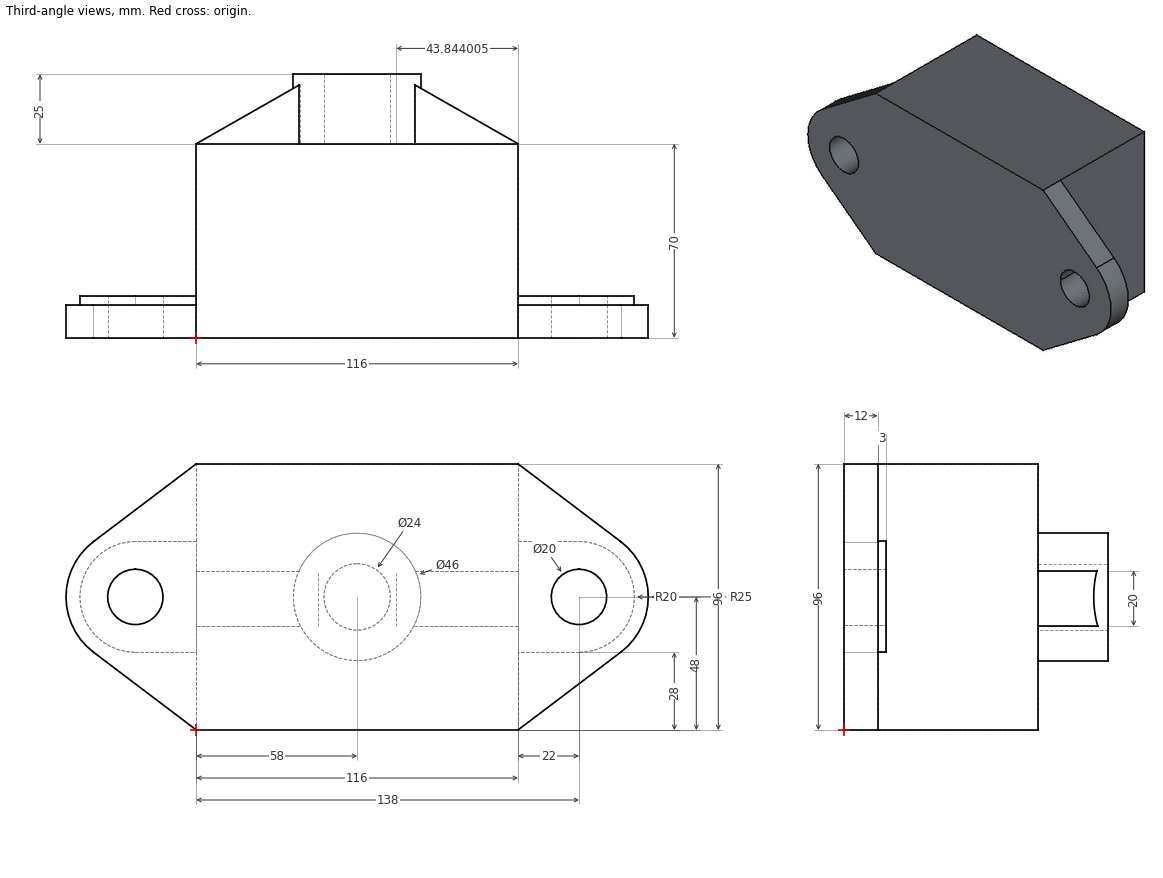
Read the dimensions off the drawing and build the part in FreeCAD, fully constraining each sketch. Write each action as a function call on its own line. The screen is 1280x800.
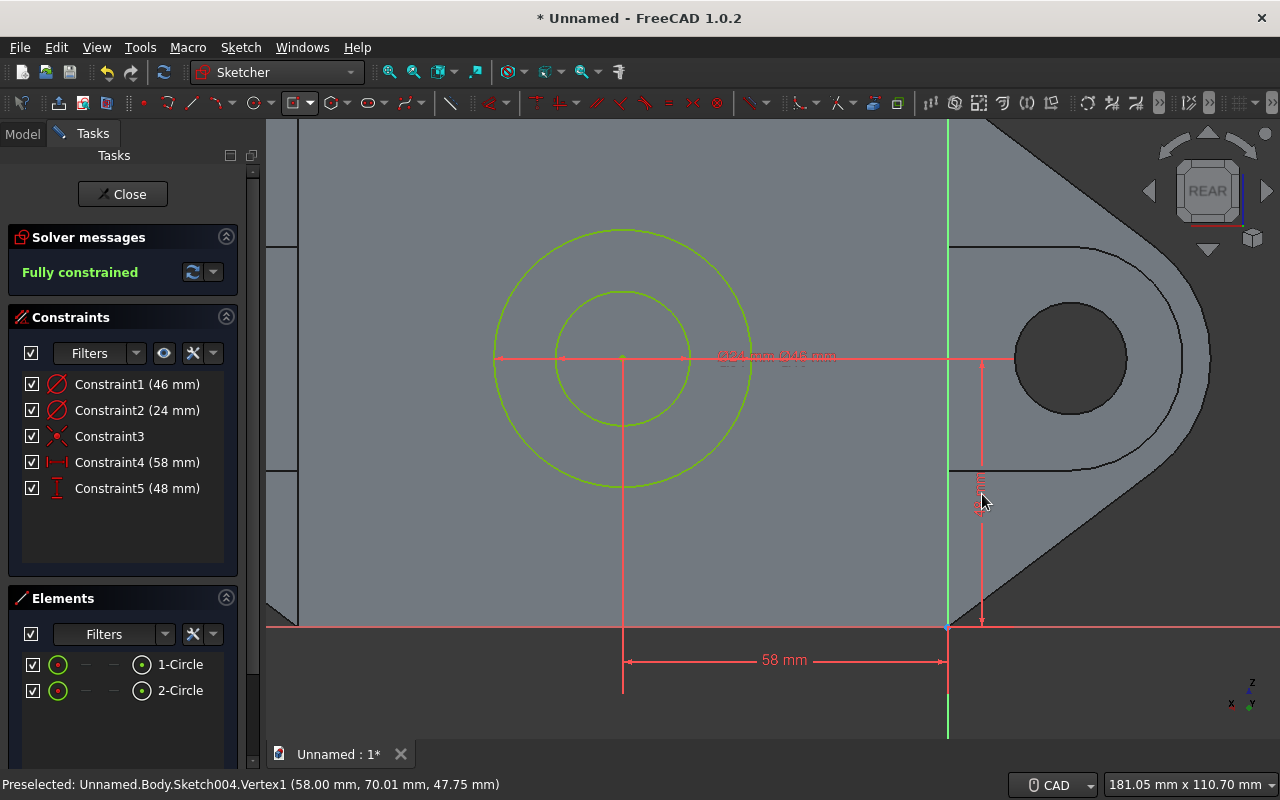
click(123, 194)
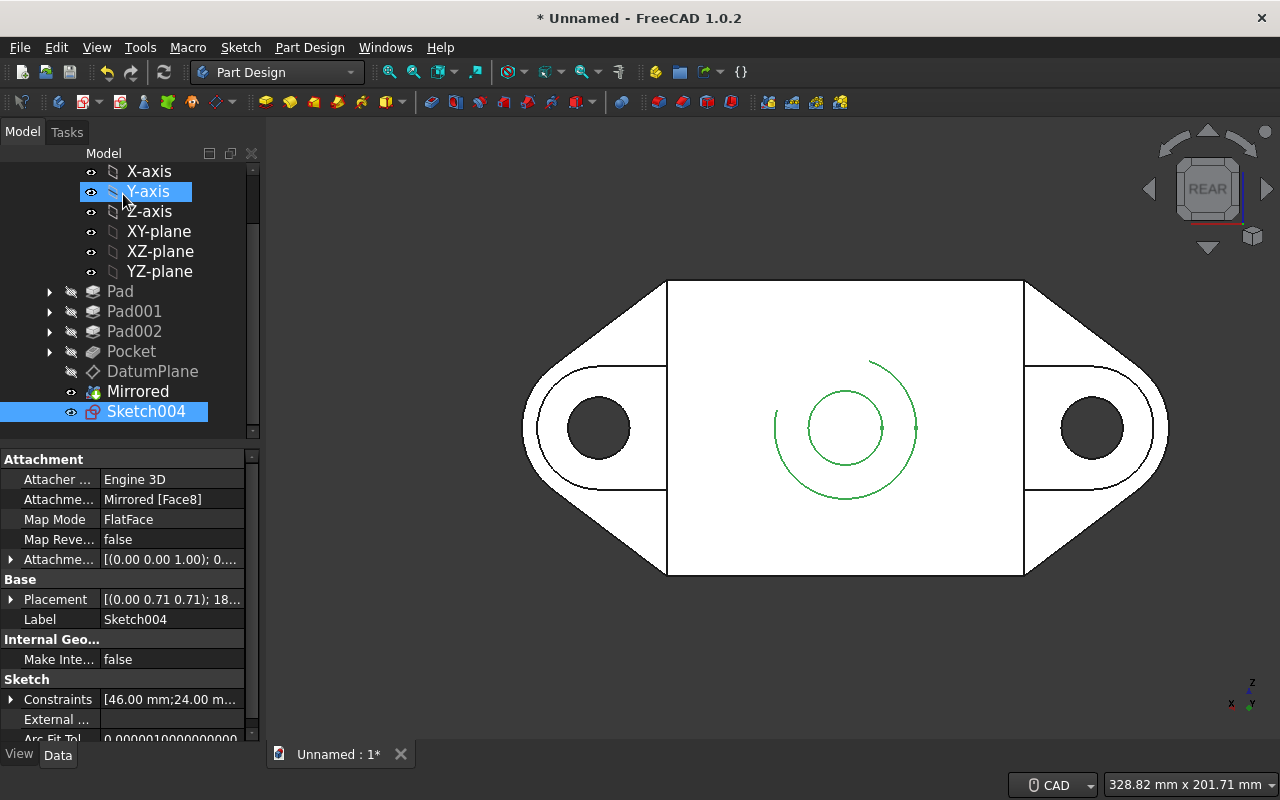
click(266, 102)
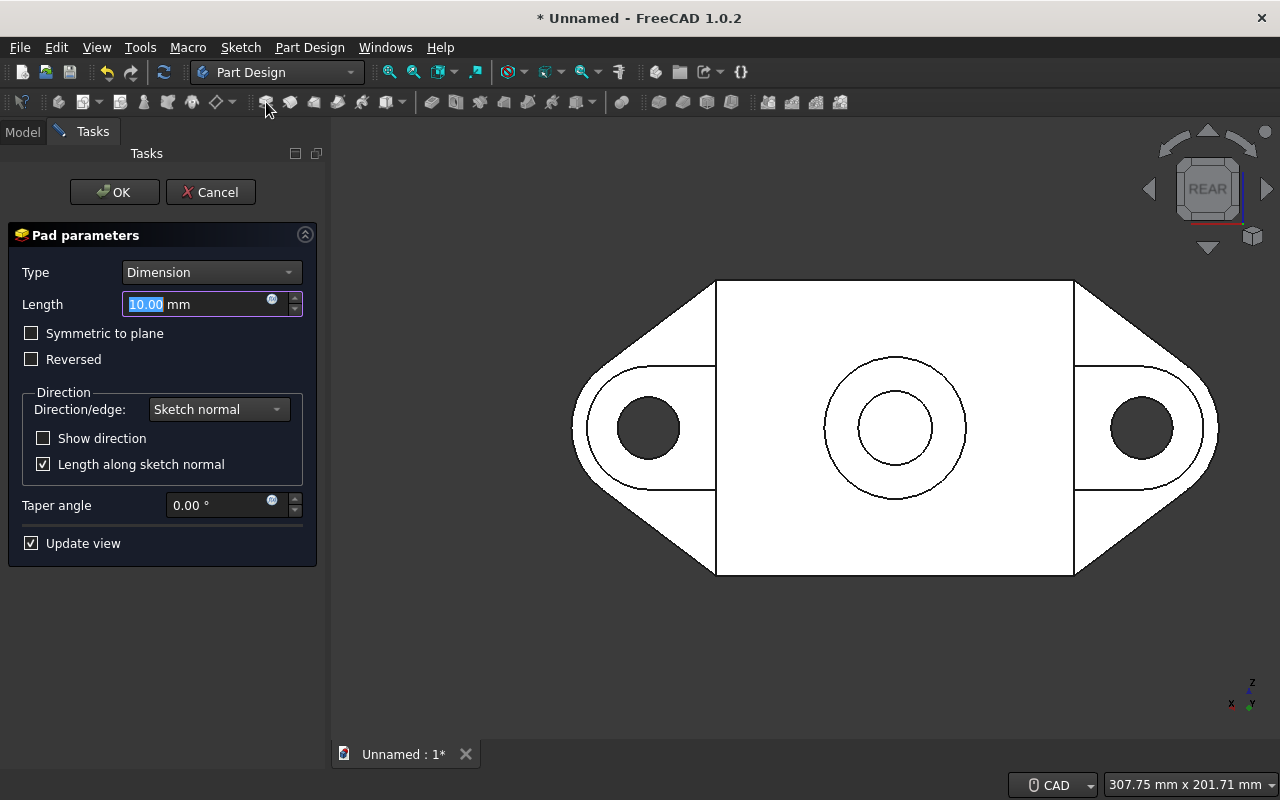
text(25)
key(Tab)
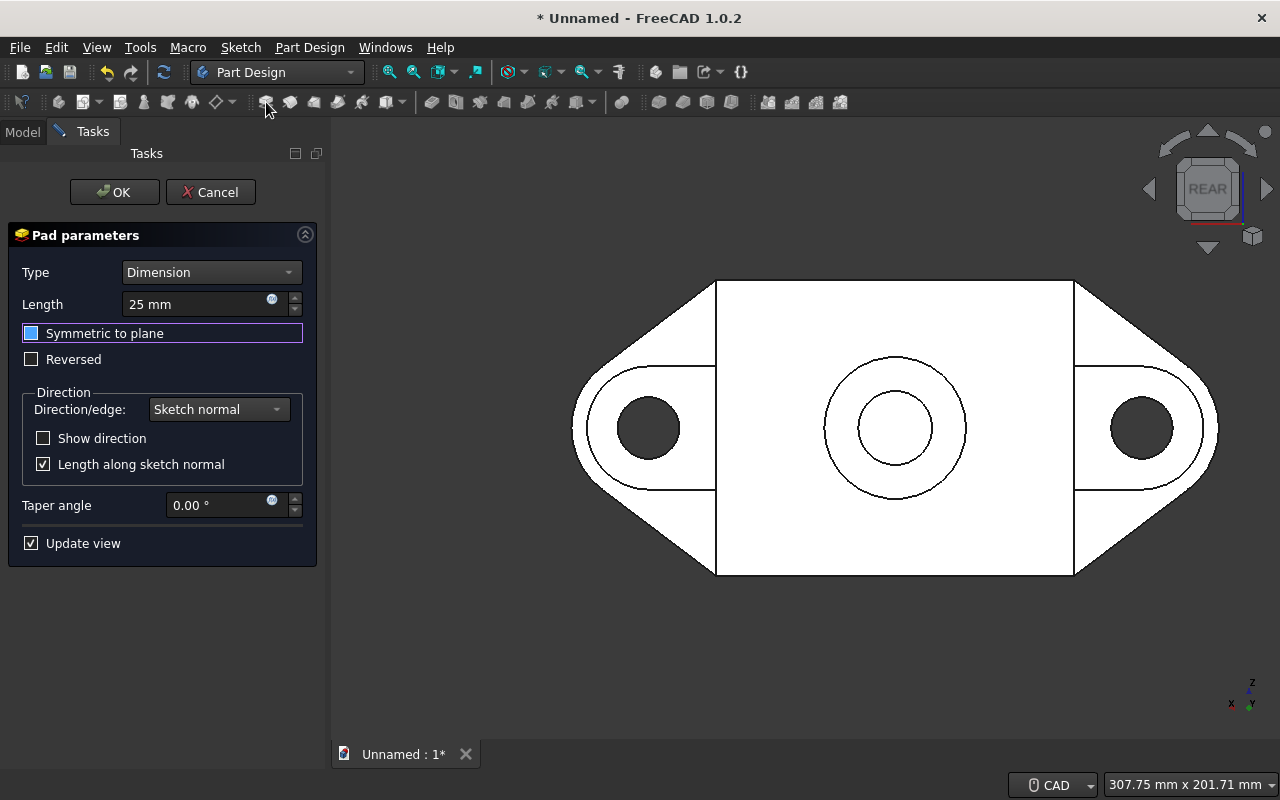
click(115, 192)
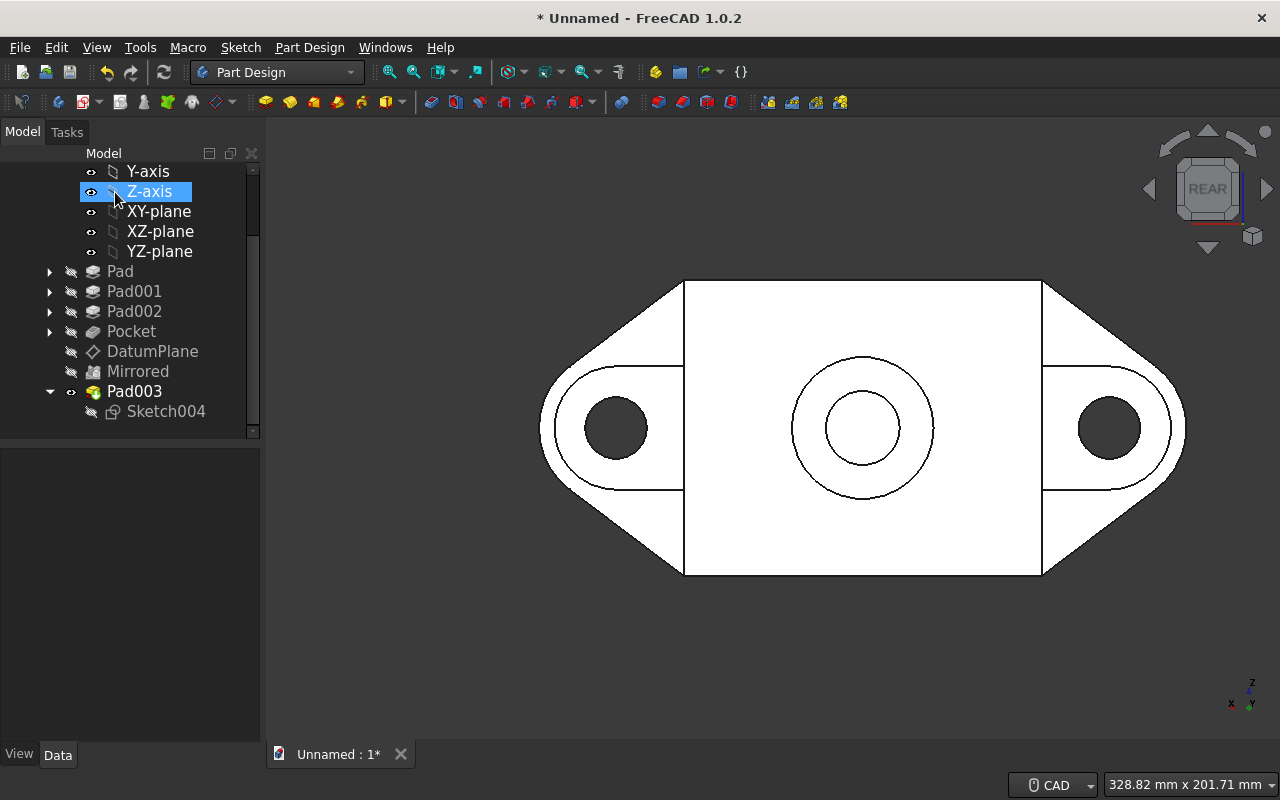
scroll(160, 287, down, 3)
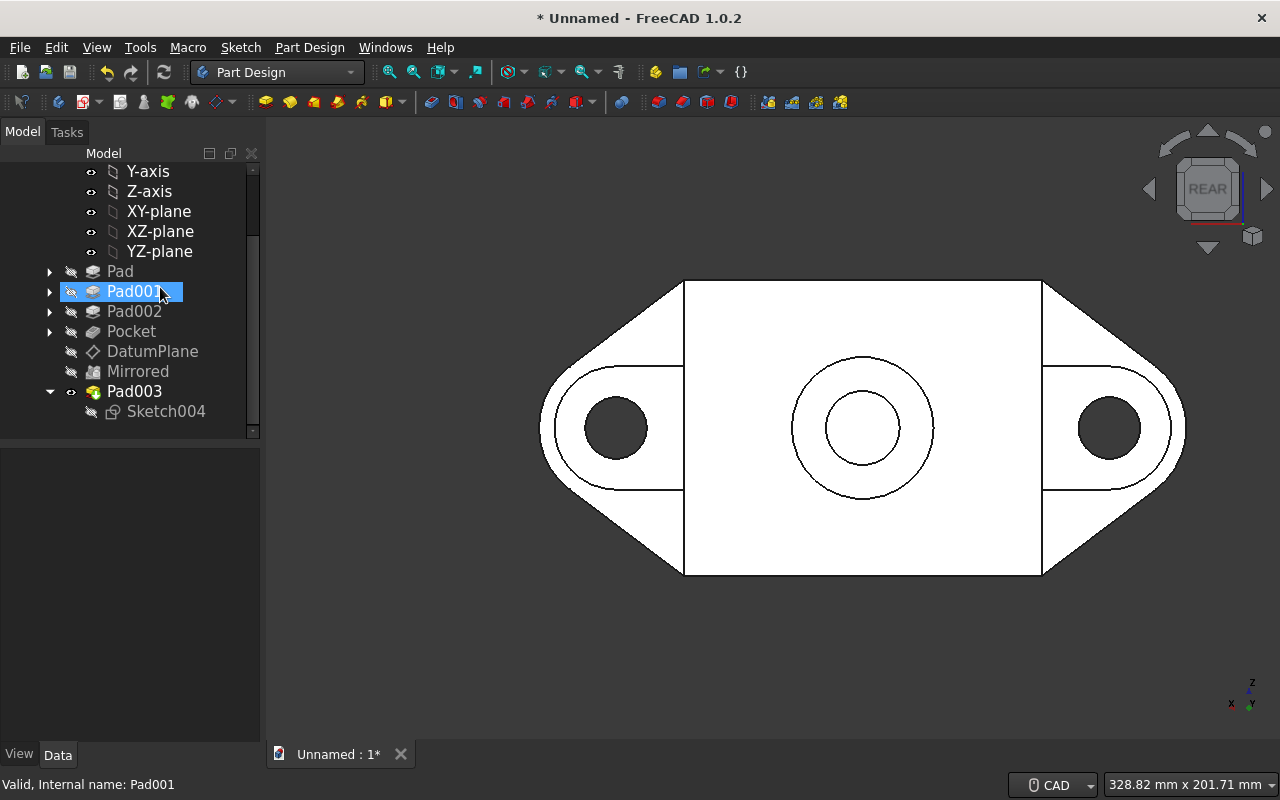
scroll(160, 287, up, 15)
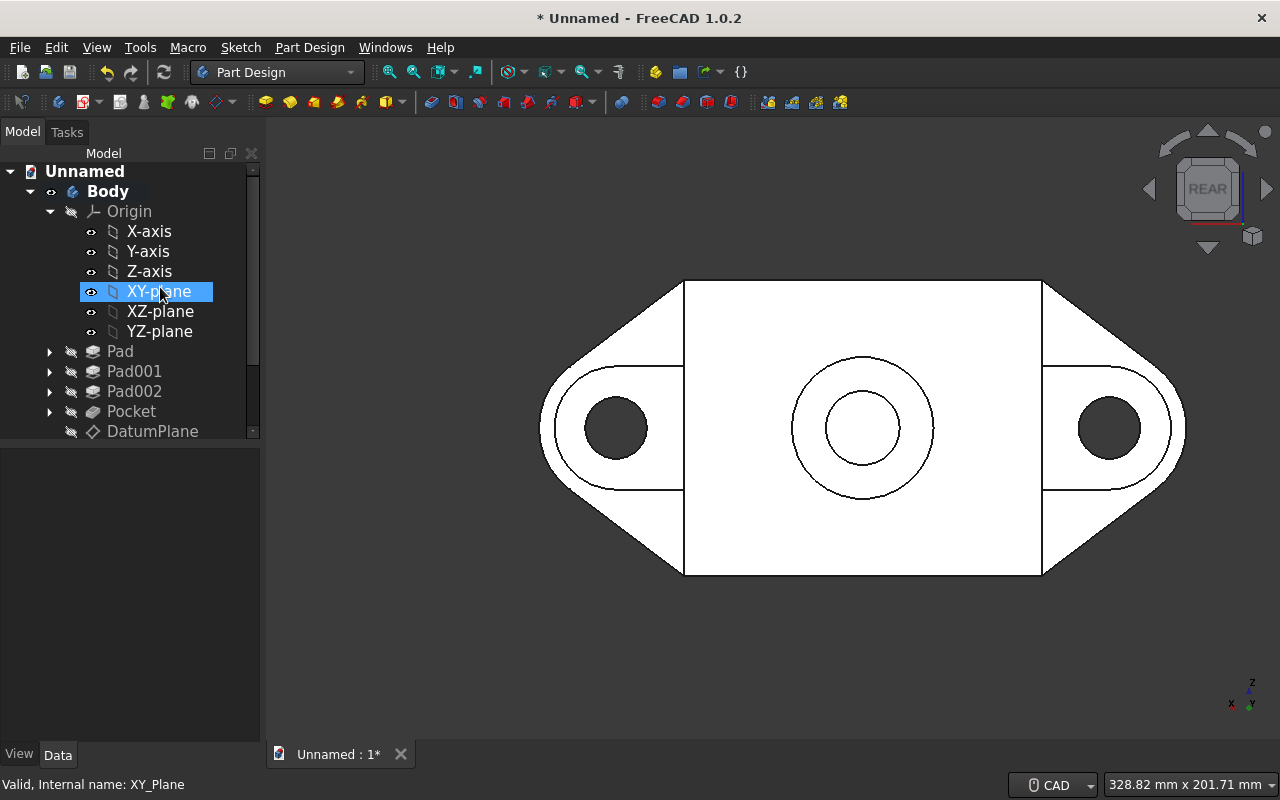
click(136, 292)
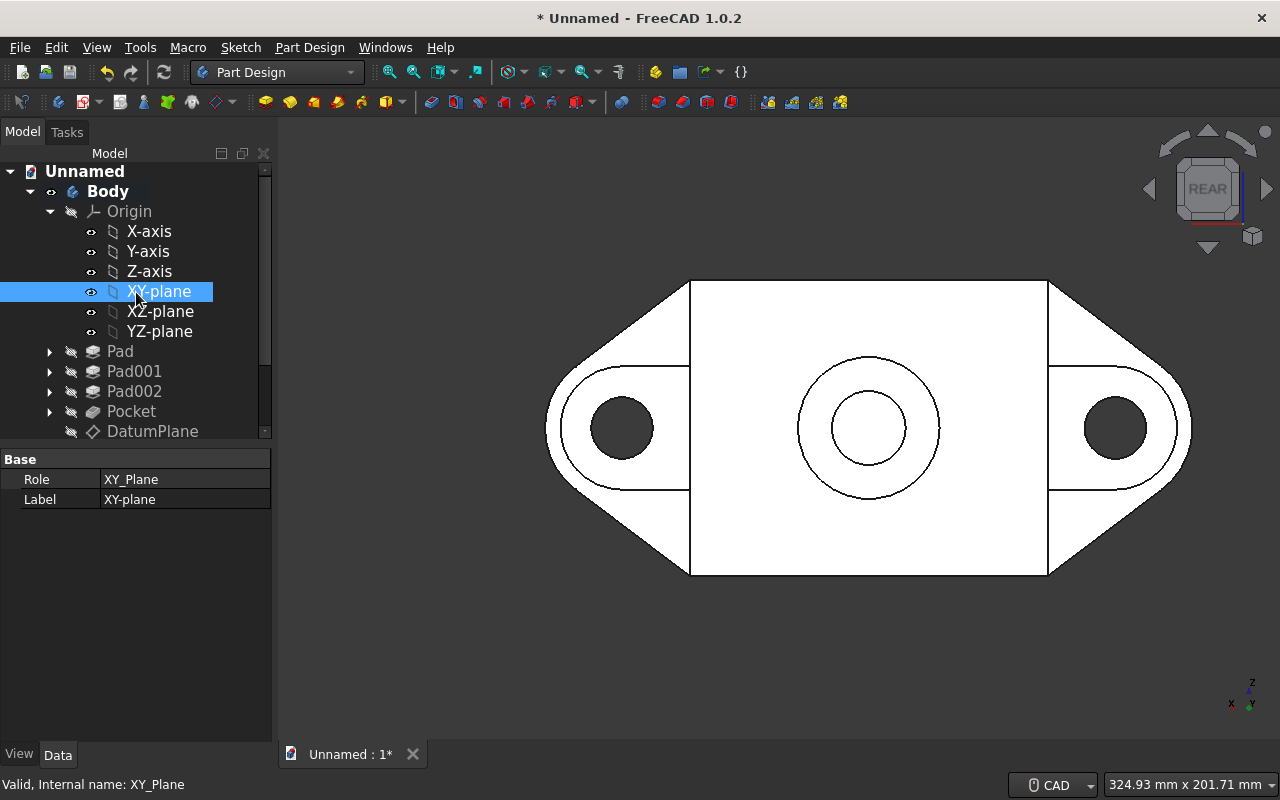
click(216, 102)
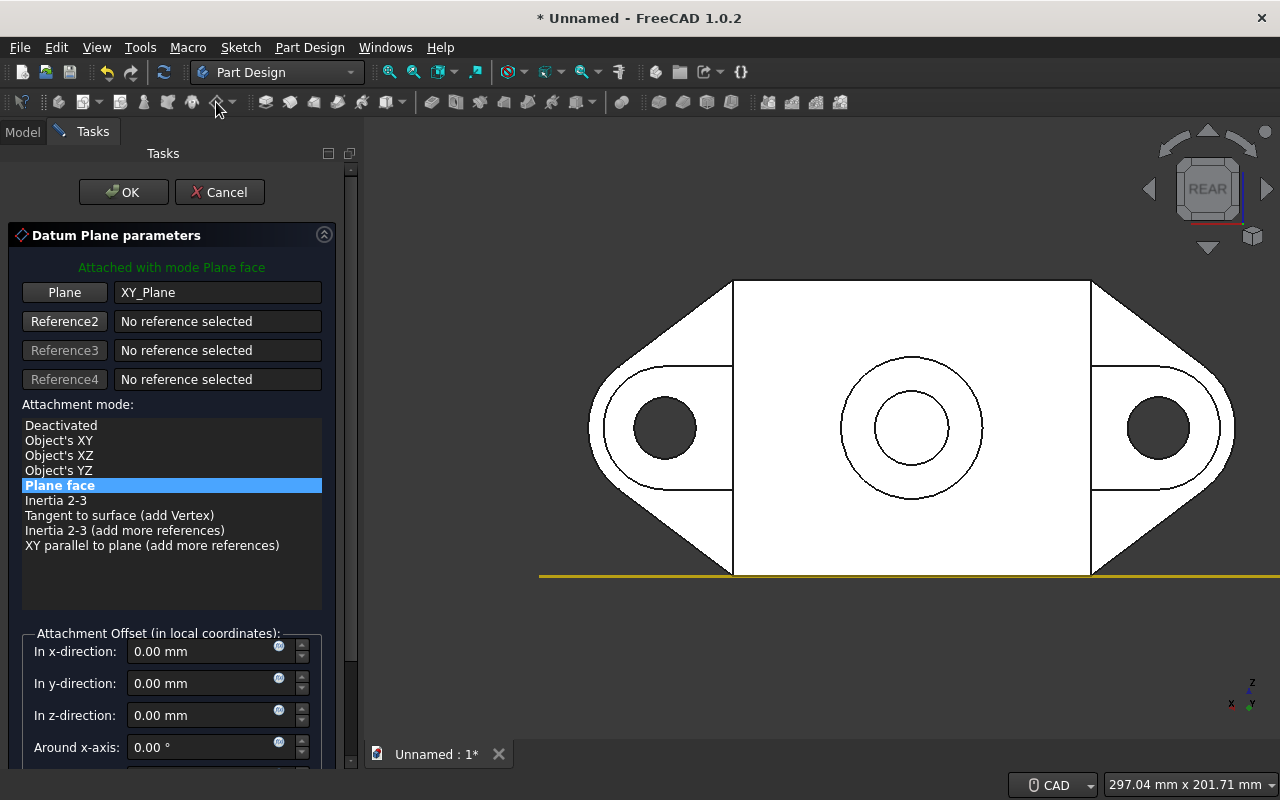
triple_click(210, 715)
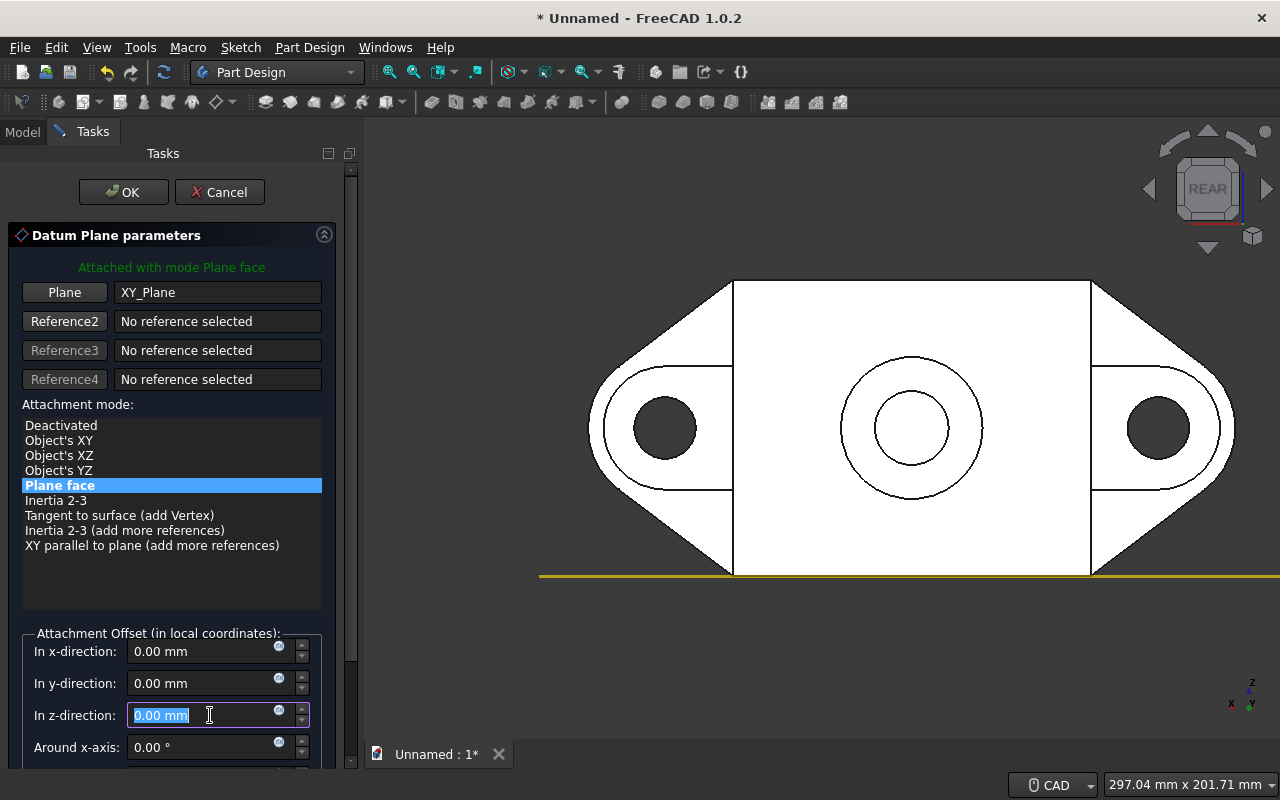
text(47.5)
key(Tab)